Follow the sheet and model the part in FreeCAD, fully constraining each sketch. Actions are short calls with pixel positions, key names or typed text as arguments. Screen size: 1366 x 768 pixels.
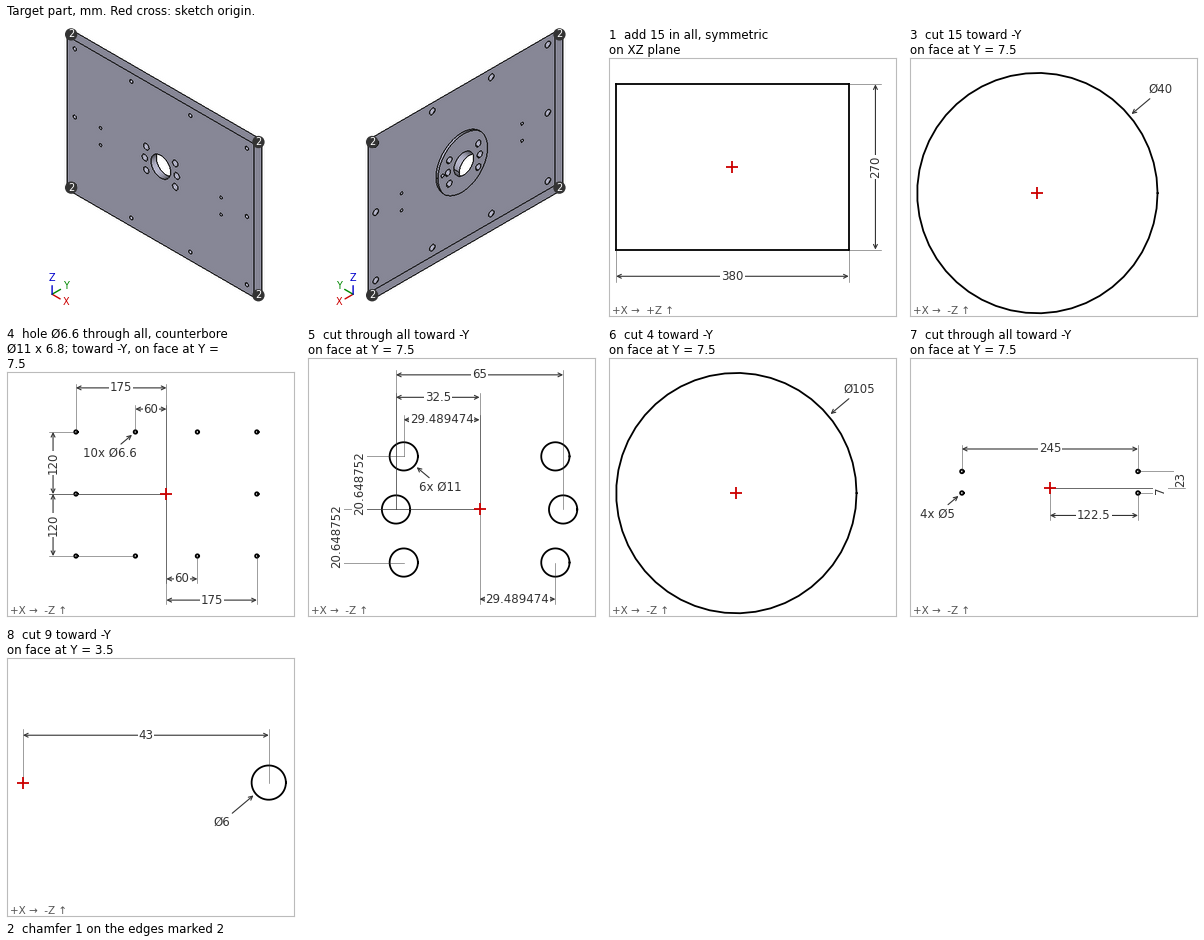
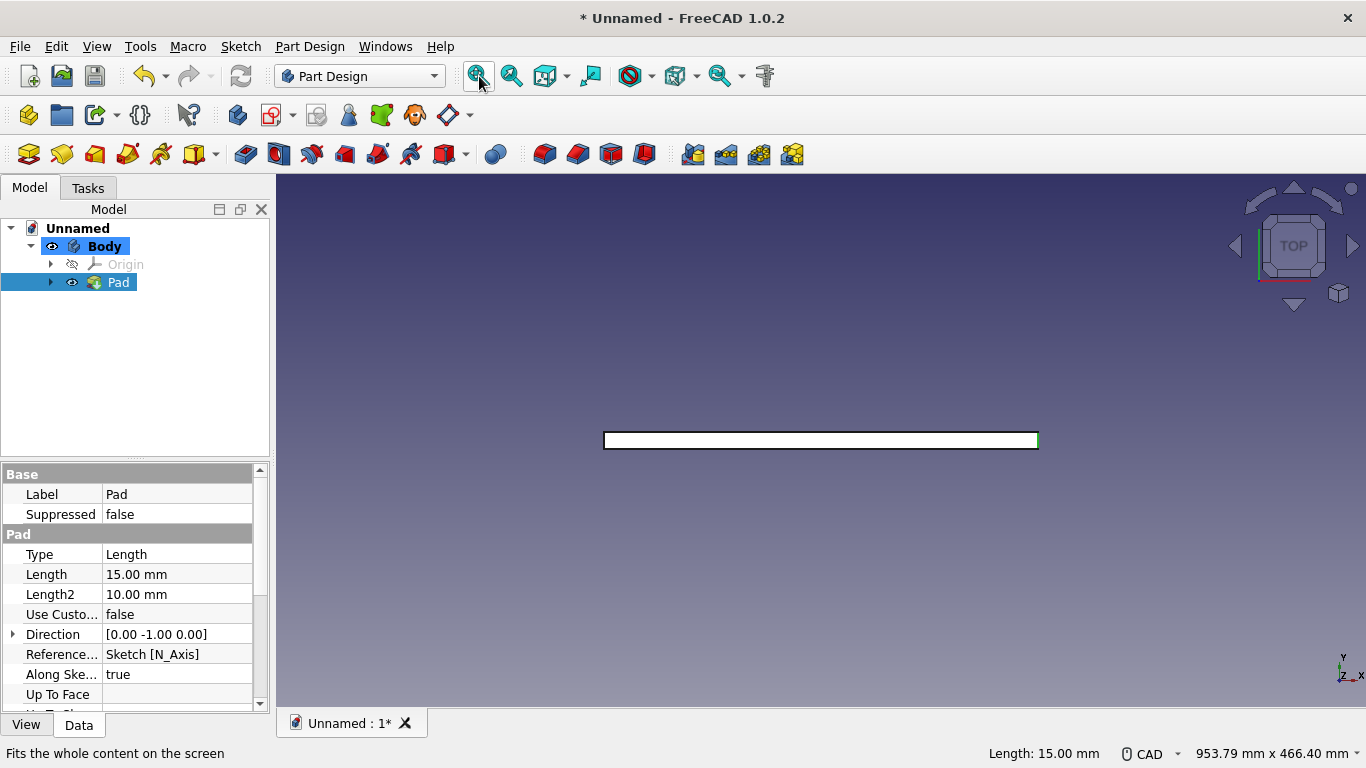
click(604, 439, ctrl)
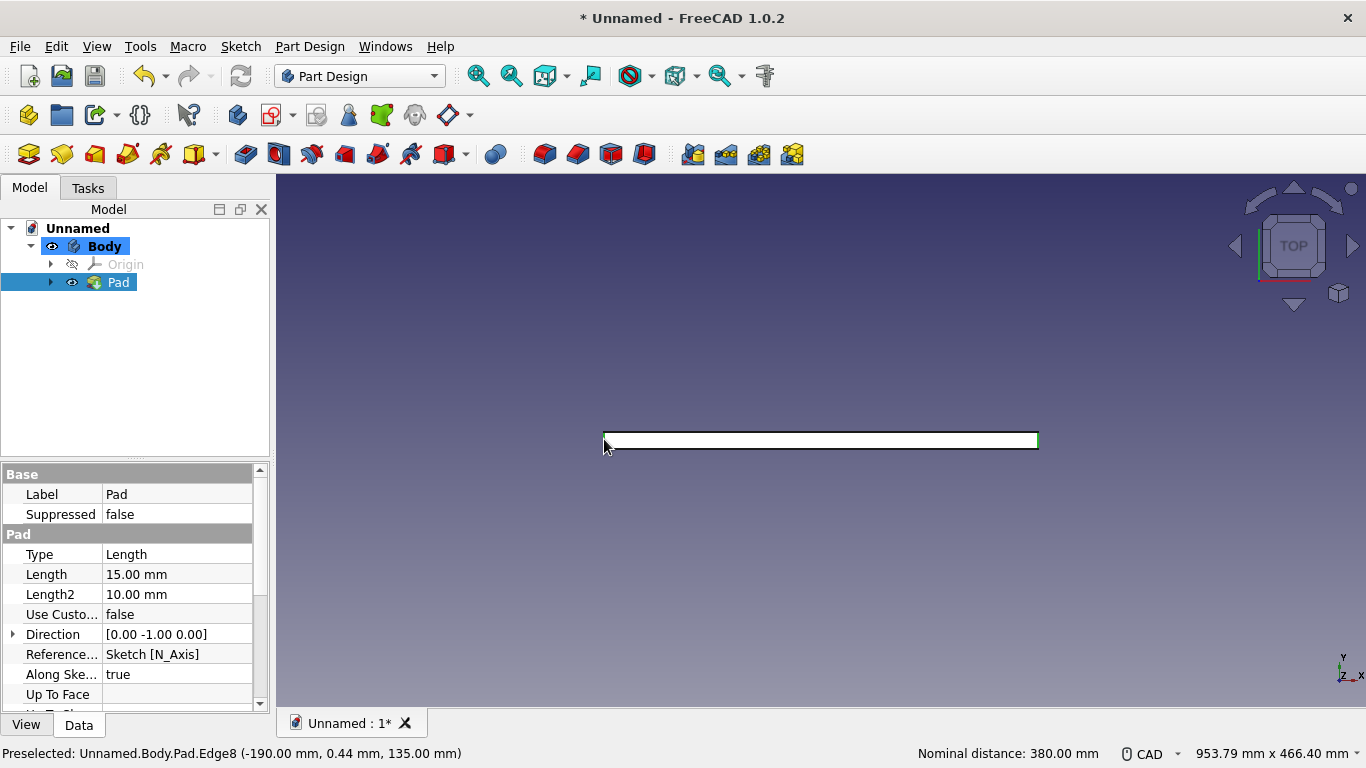
scroll(604, 439, up, 5)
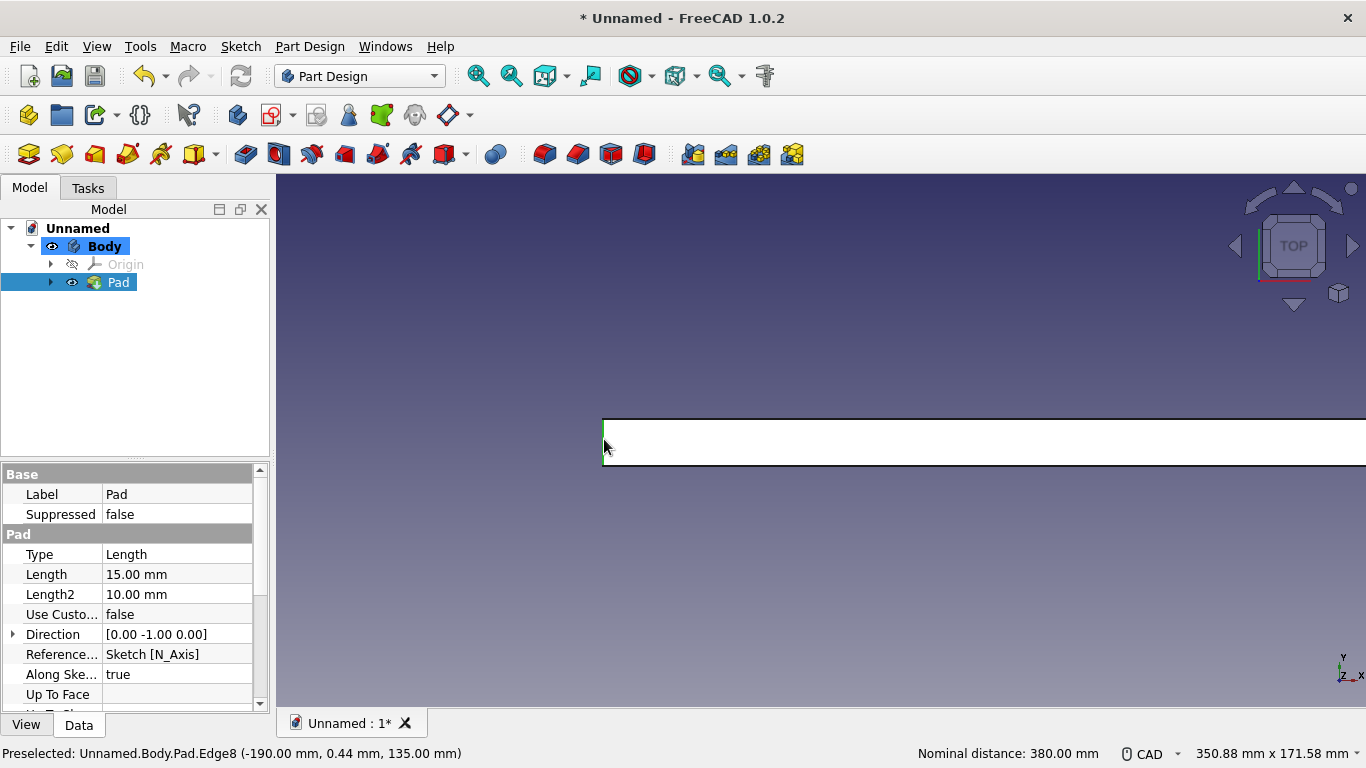
click(479, 76)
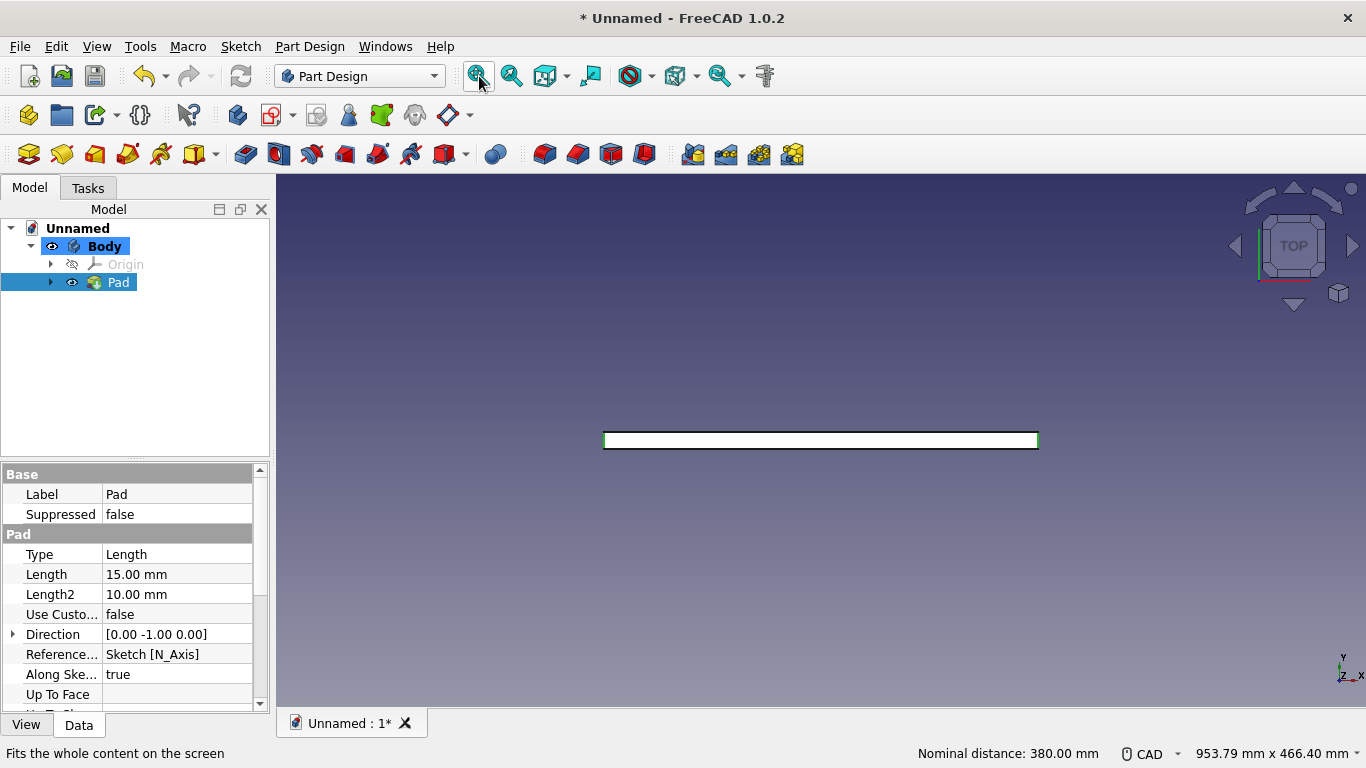
key(1)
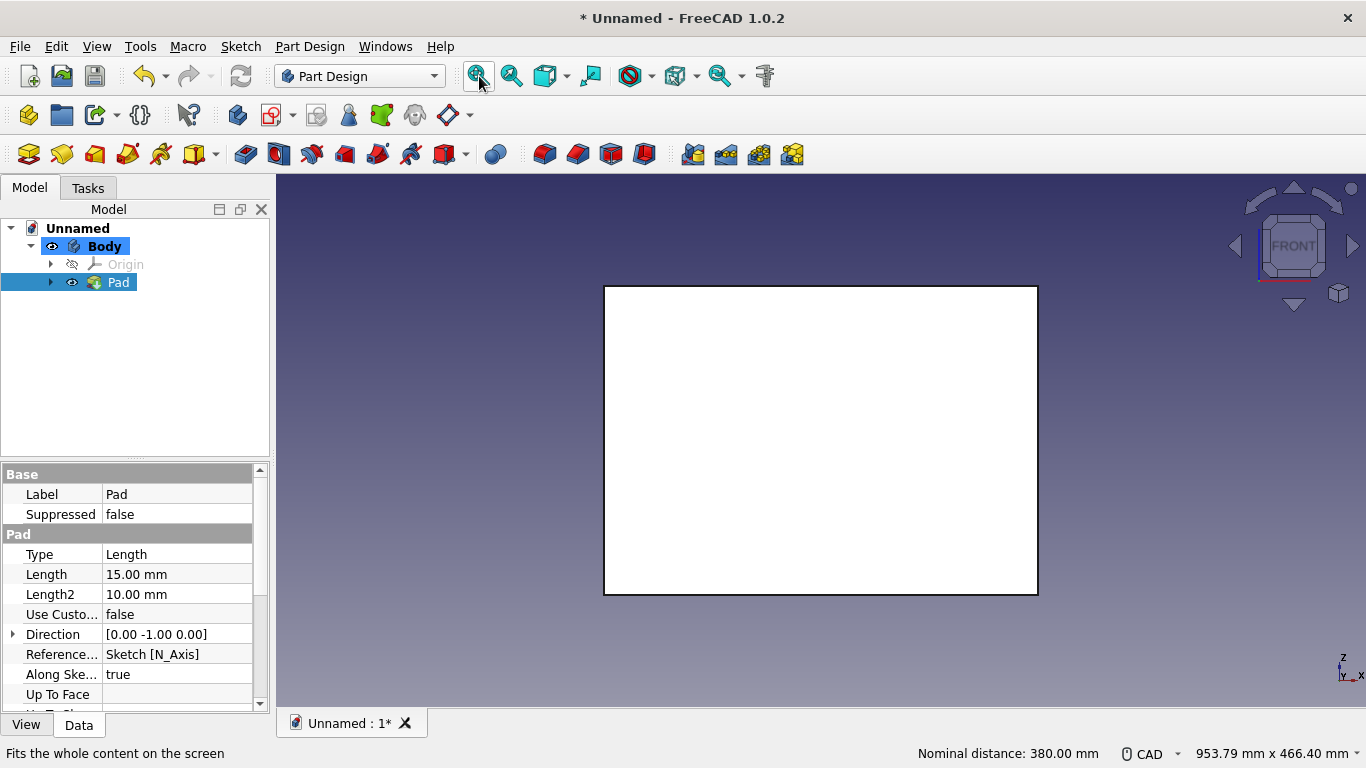
scroll(604, 594, up, 5)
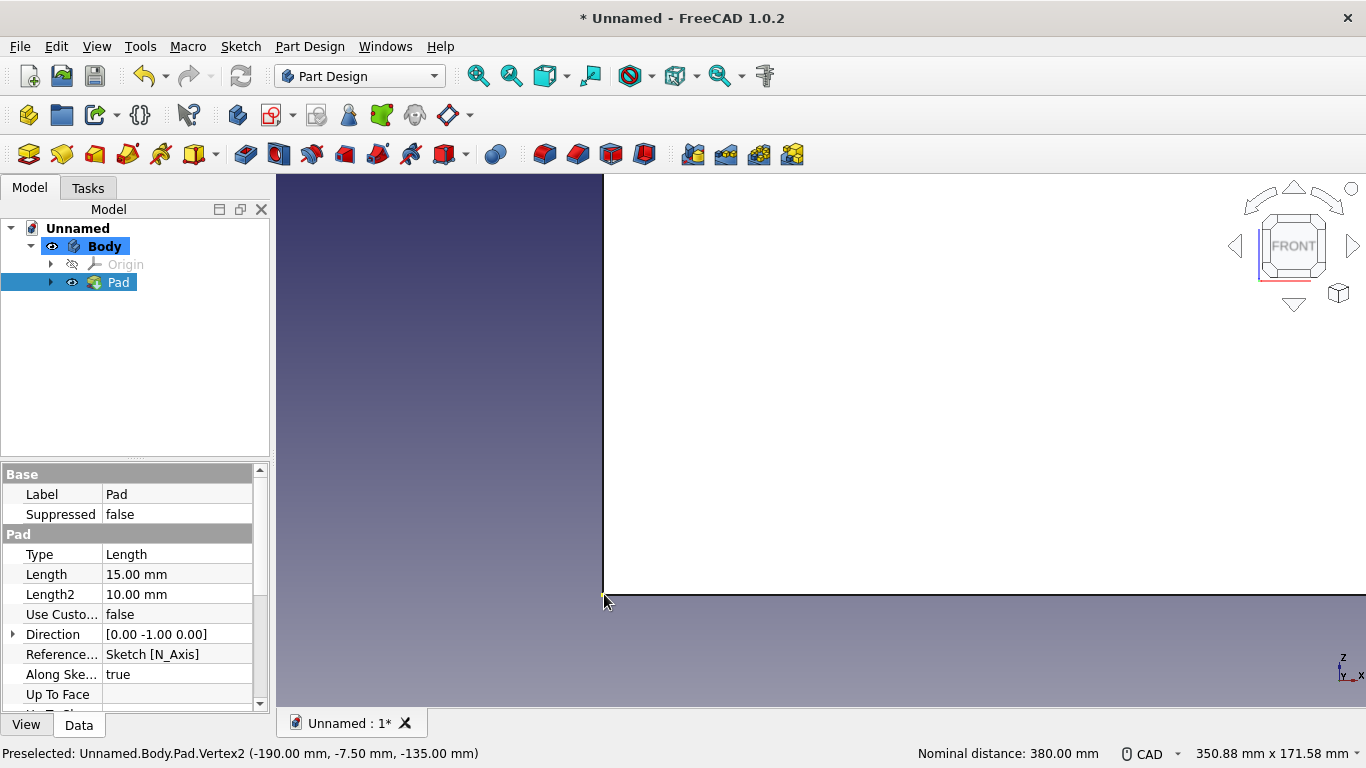
click(479, 76)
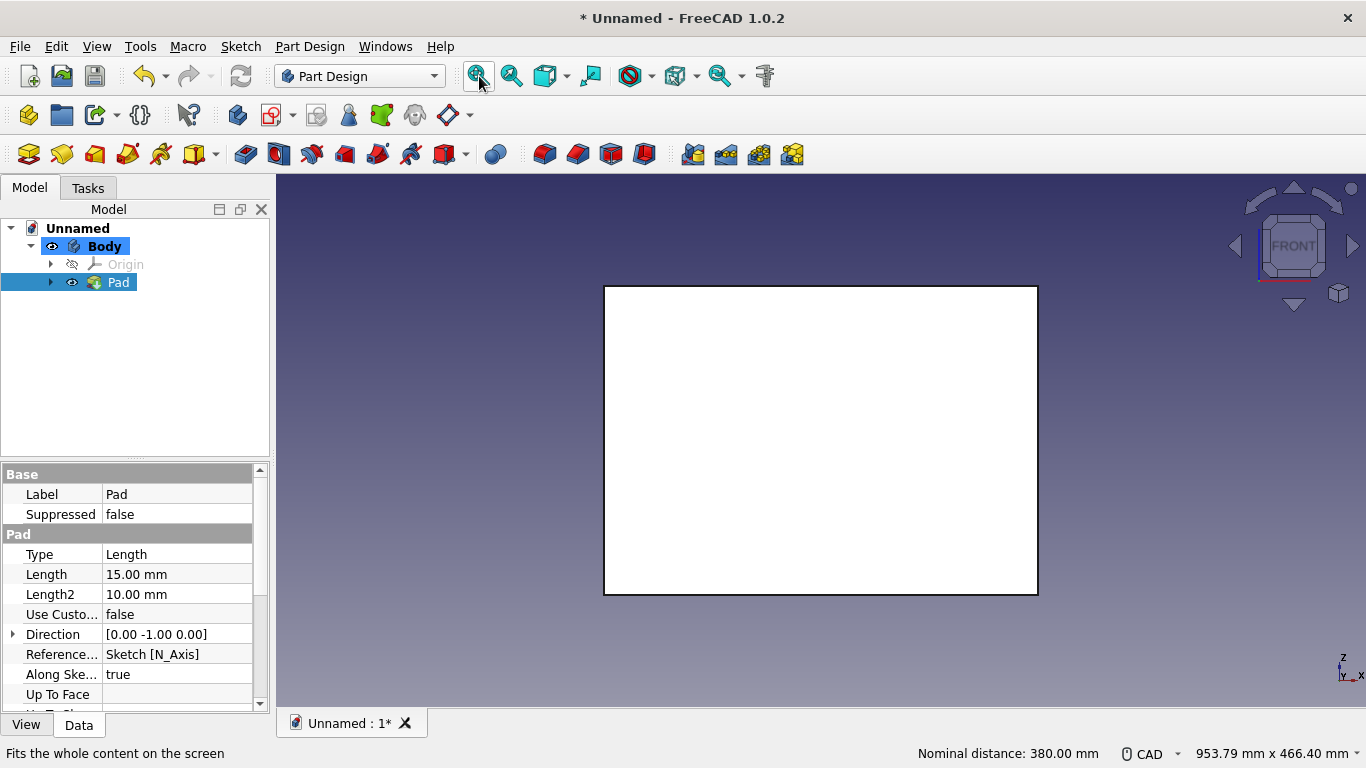
key(3)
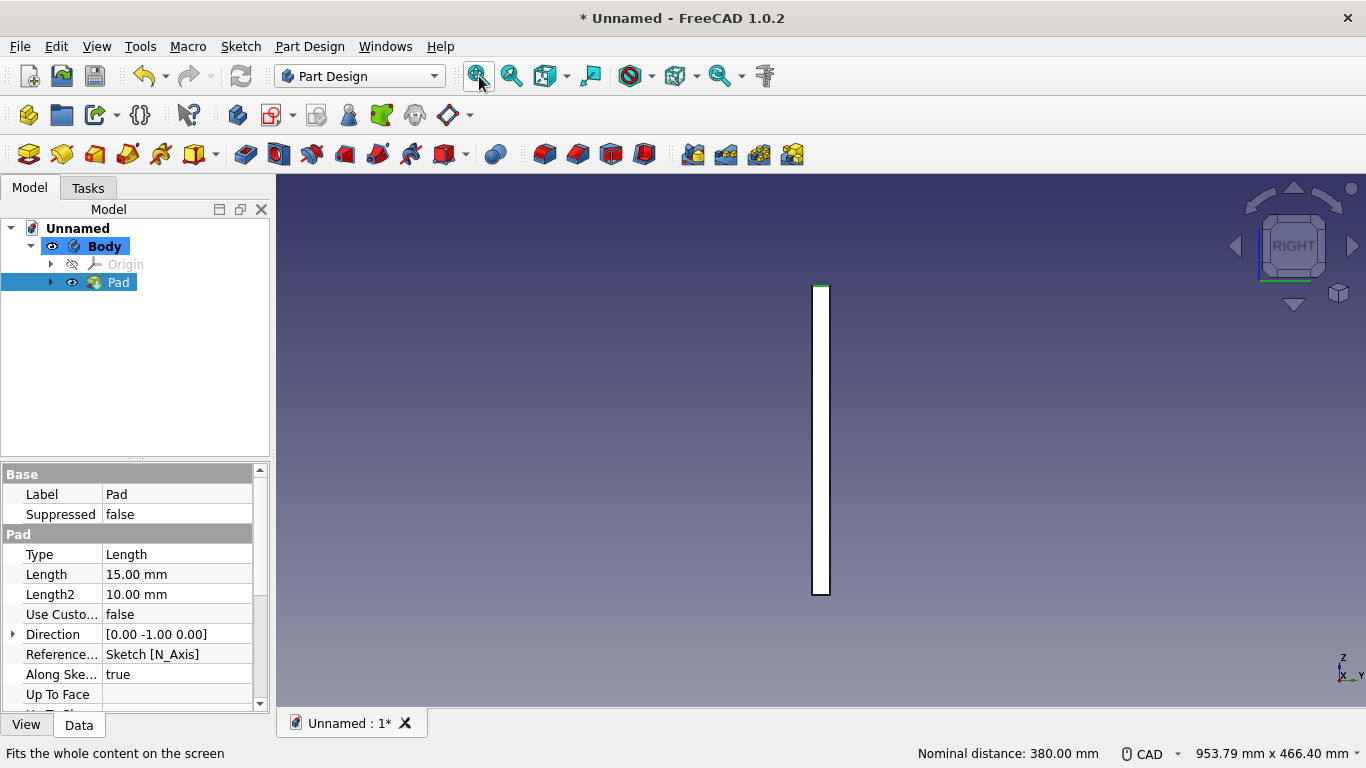
click(821, 594, ctrl)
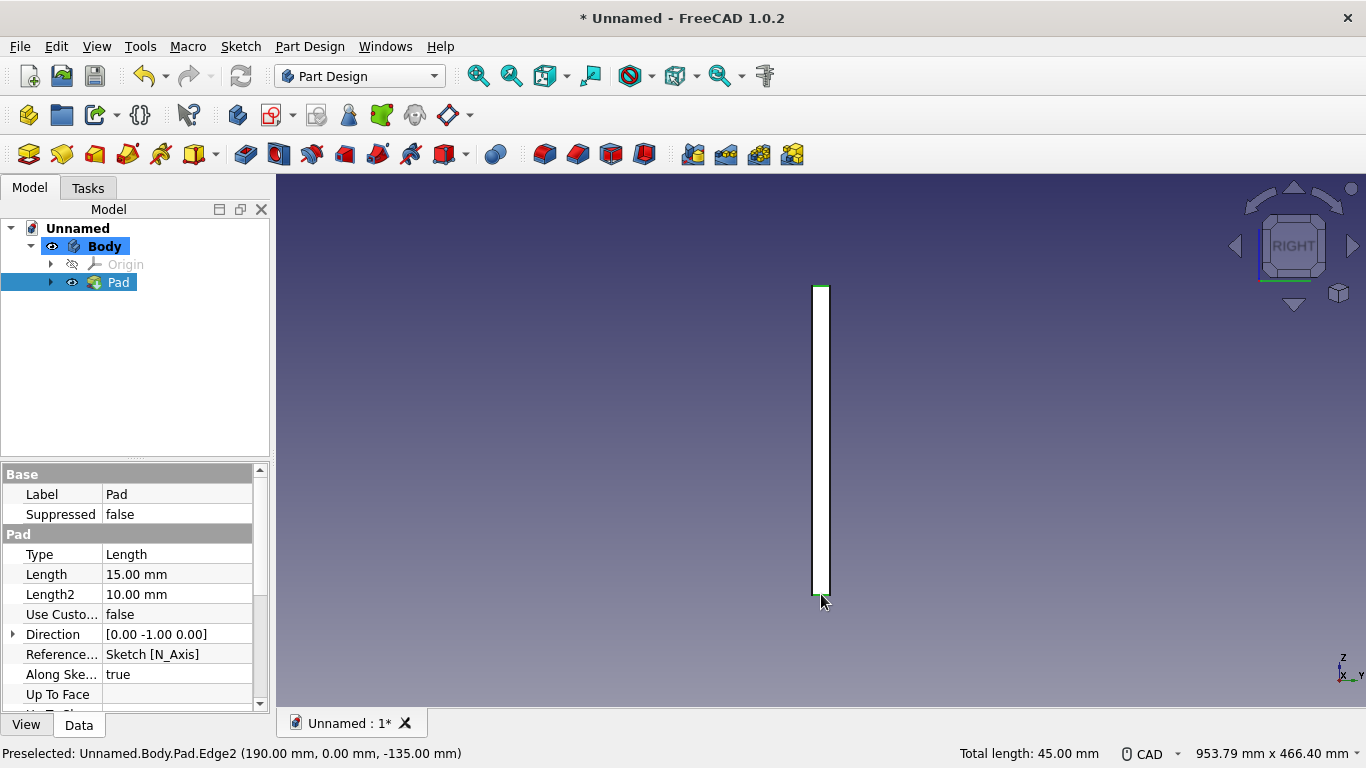
scroll(821, 594, up, 5)